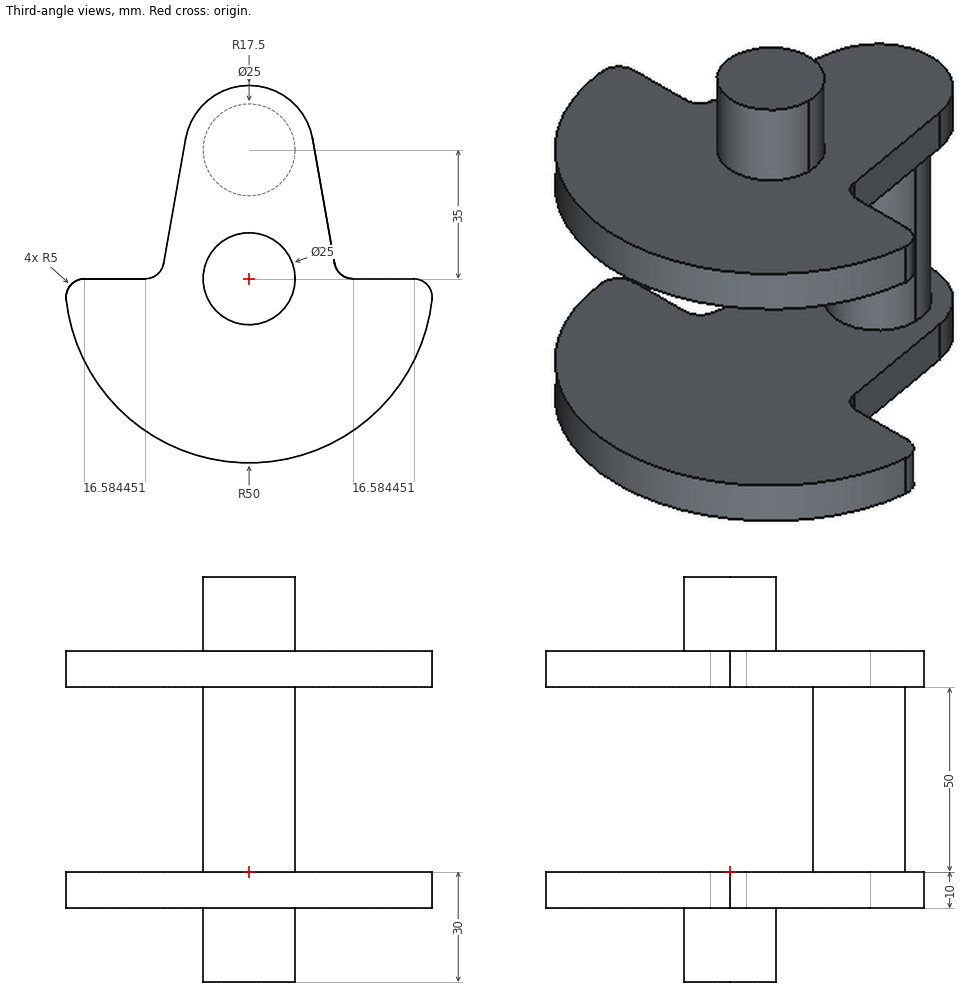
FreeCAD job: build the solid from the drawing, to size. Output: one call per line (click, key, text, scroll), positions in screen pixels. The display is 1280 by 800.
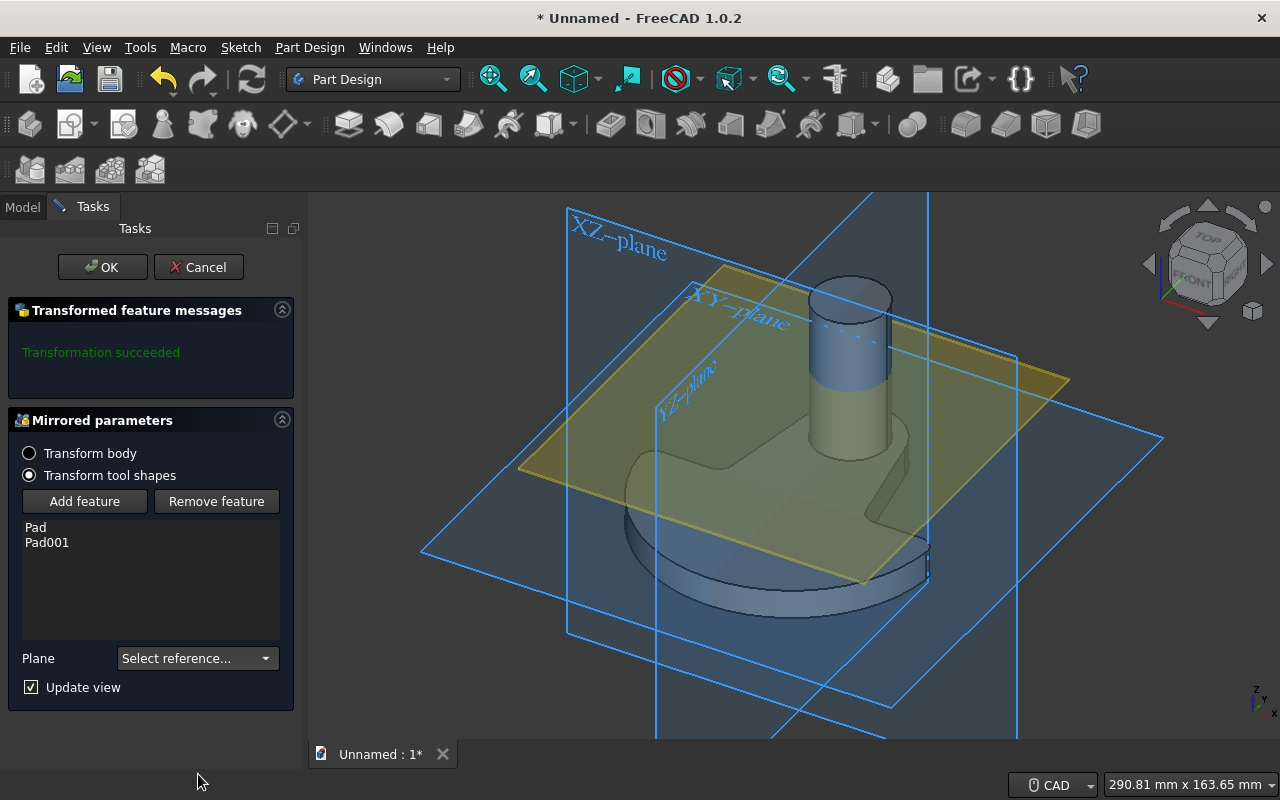
click(23, 206)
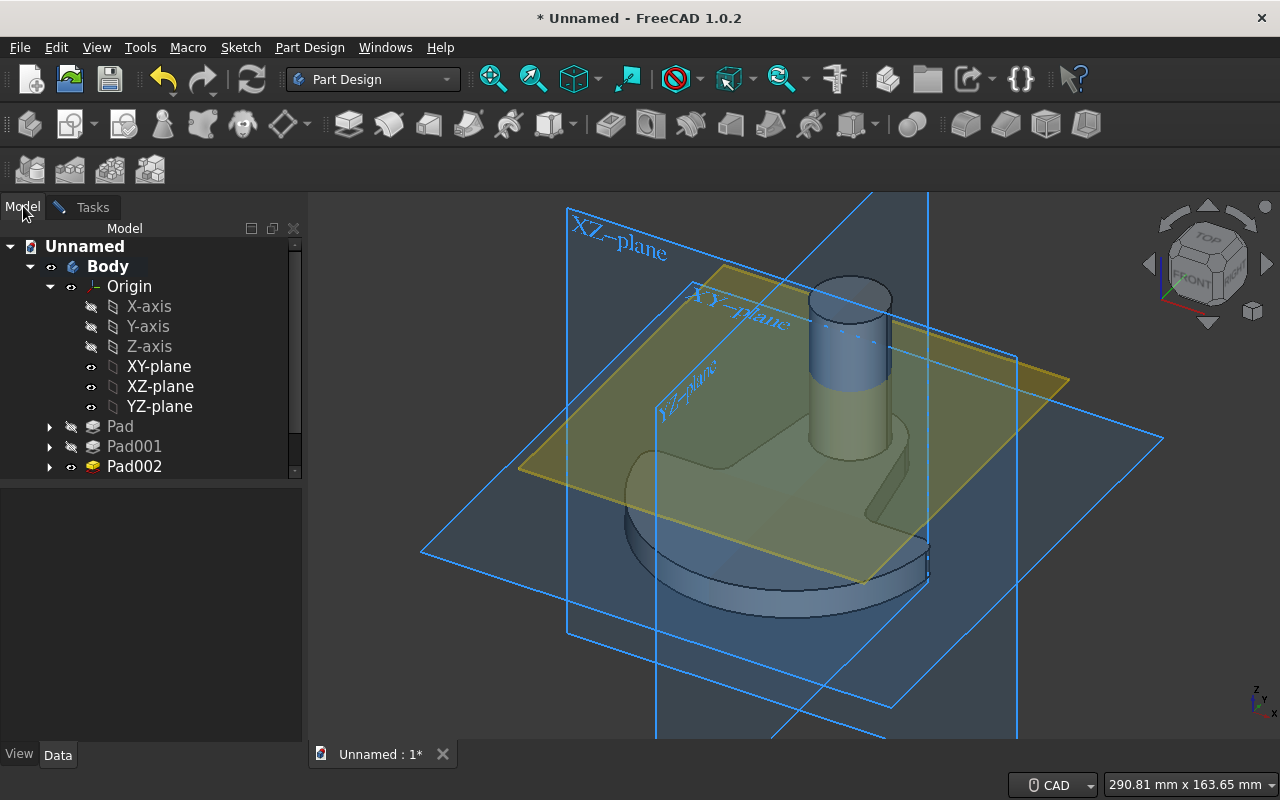
scroll(100, 362, down, 3)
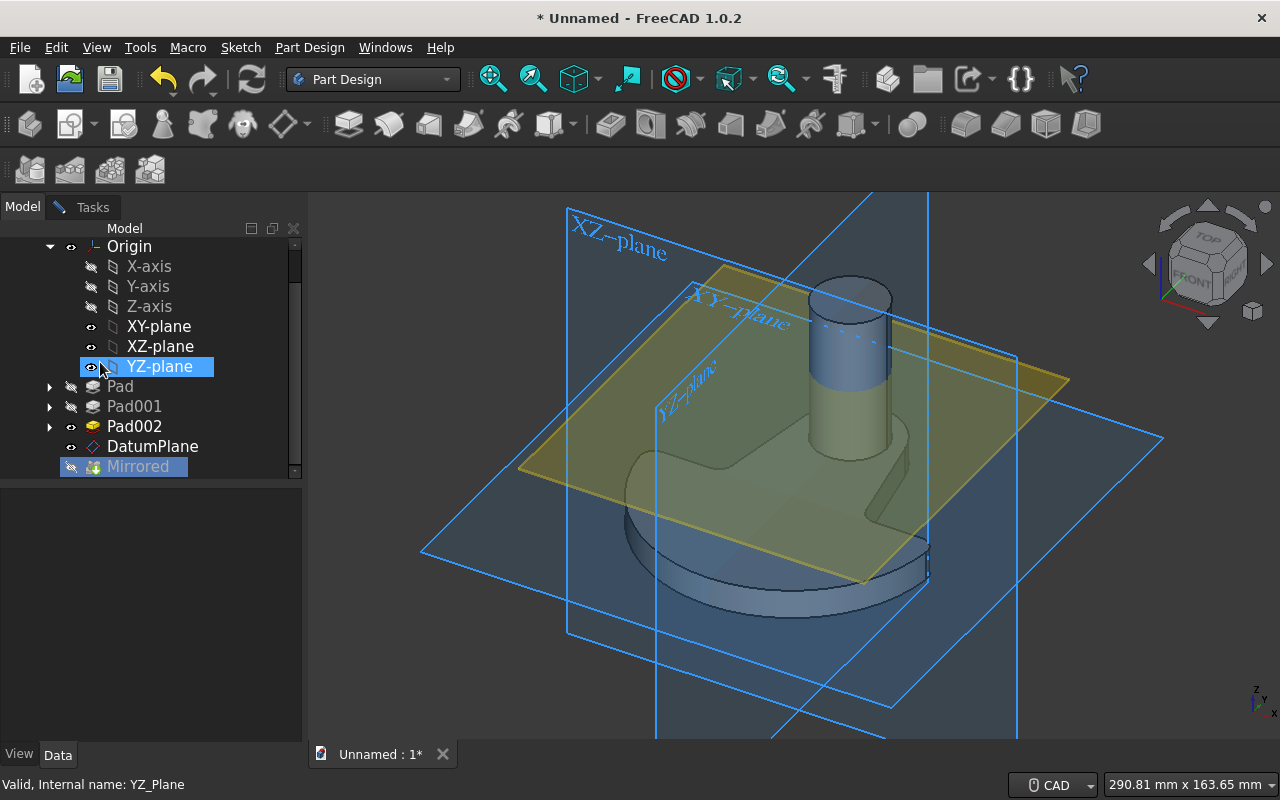
click(116, 447)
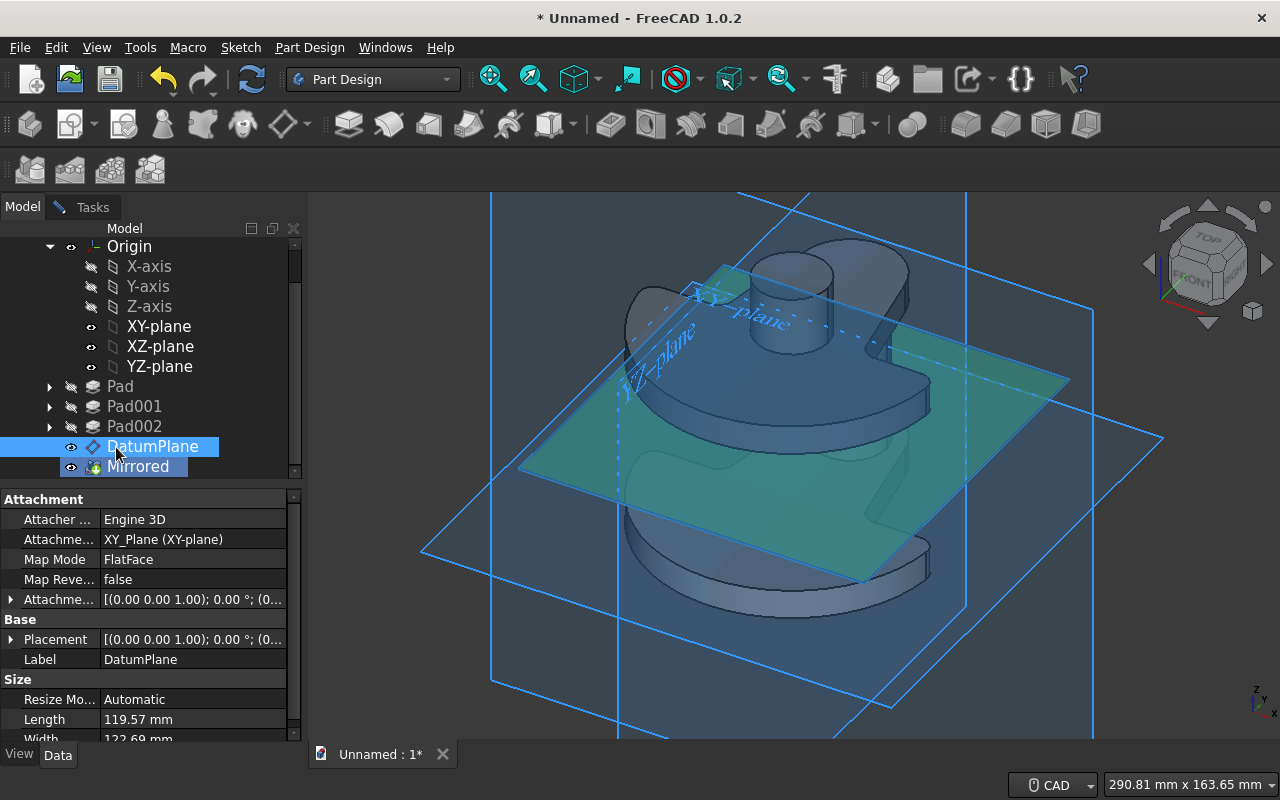
click(84, 206)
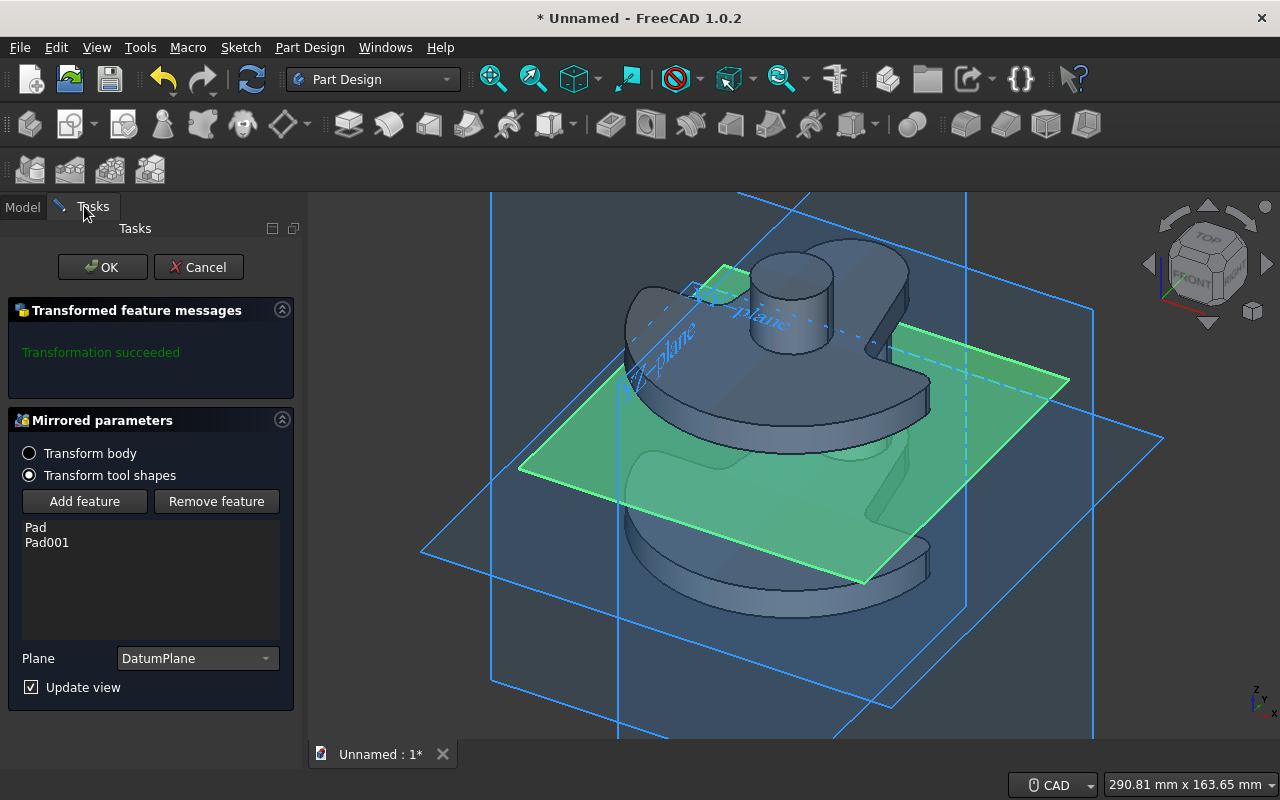
click(103, 267)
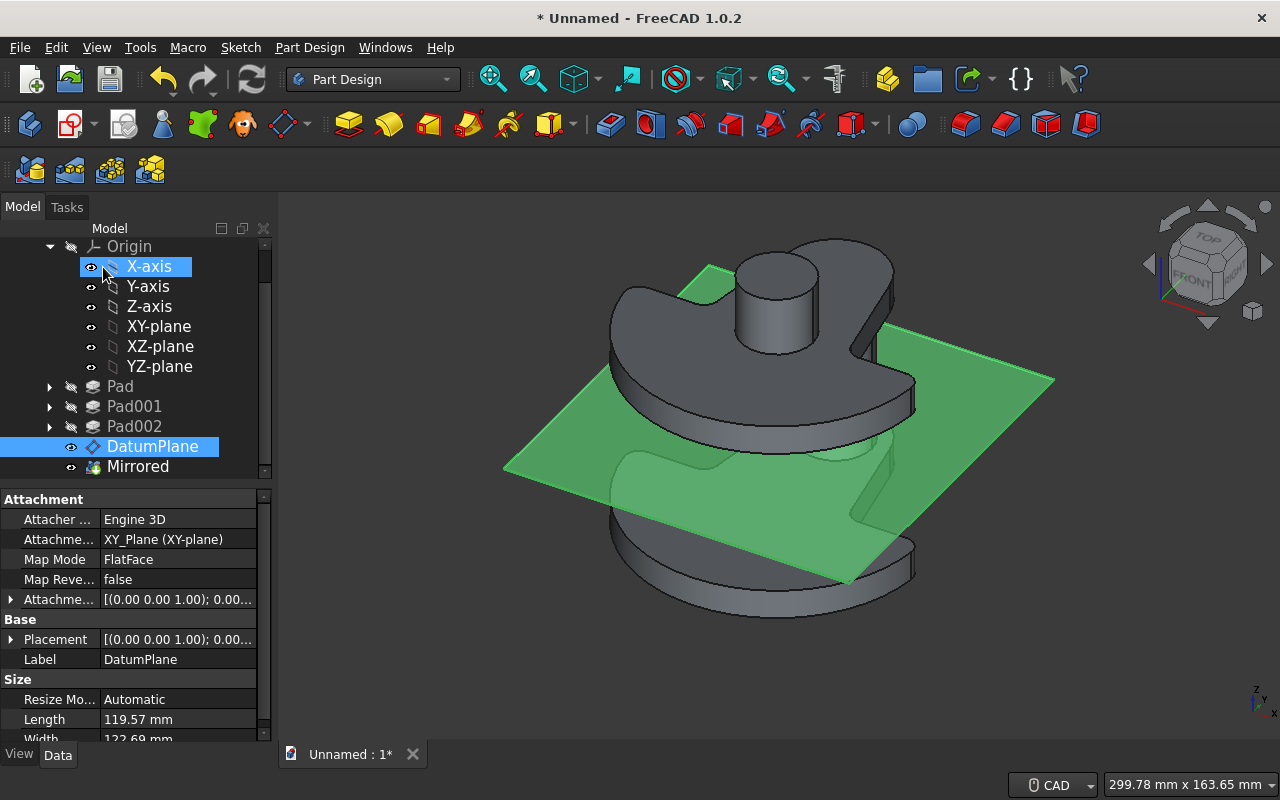
click(116, 447)
key(space)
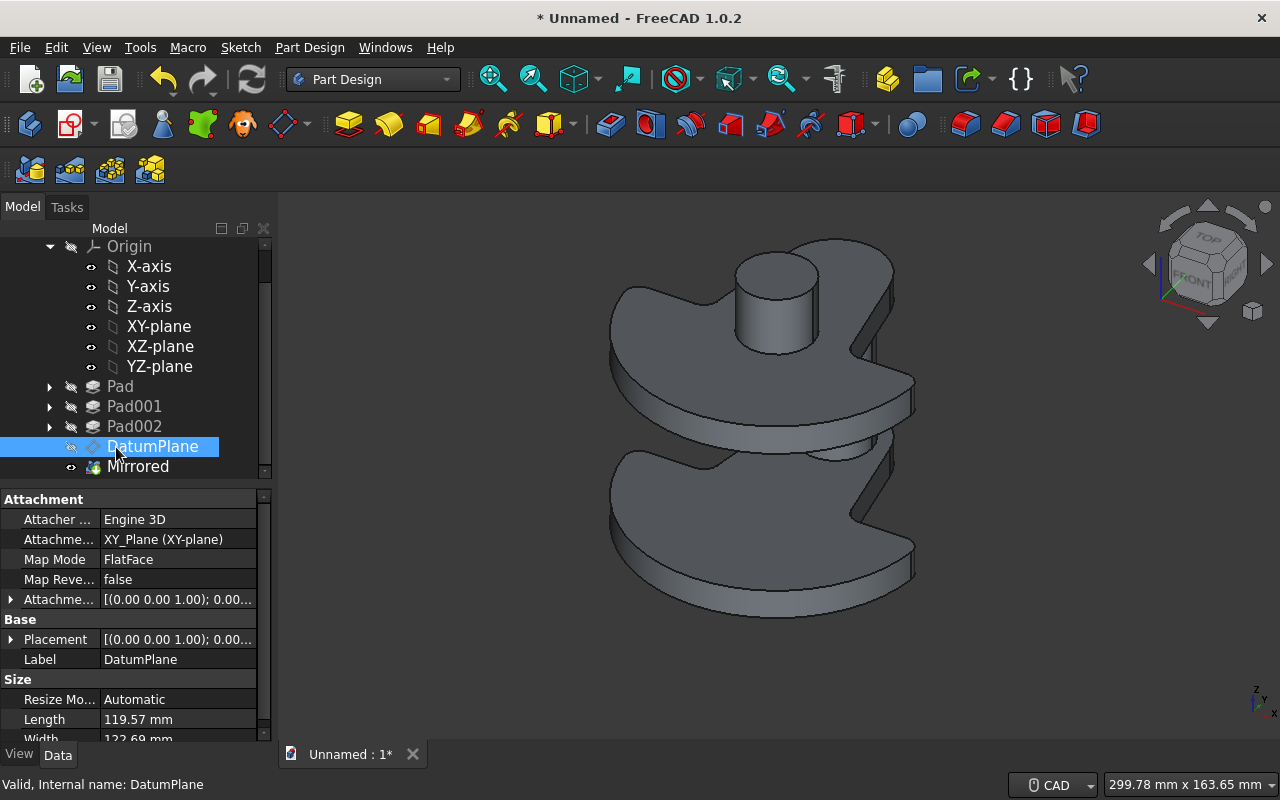
key(0)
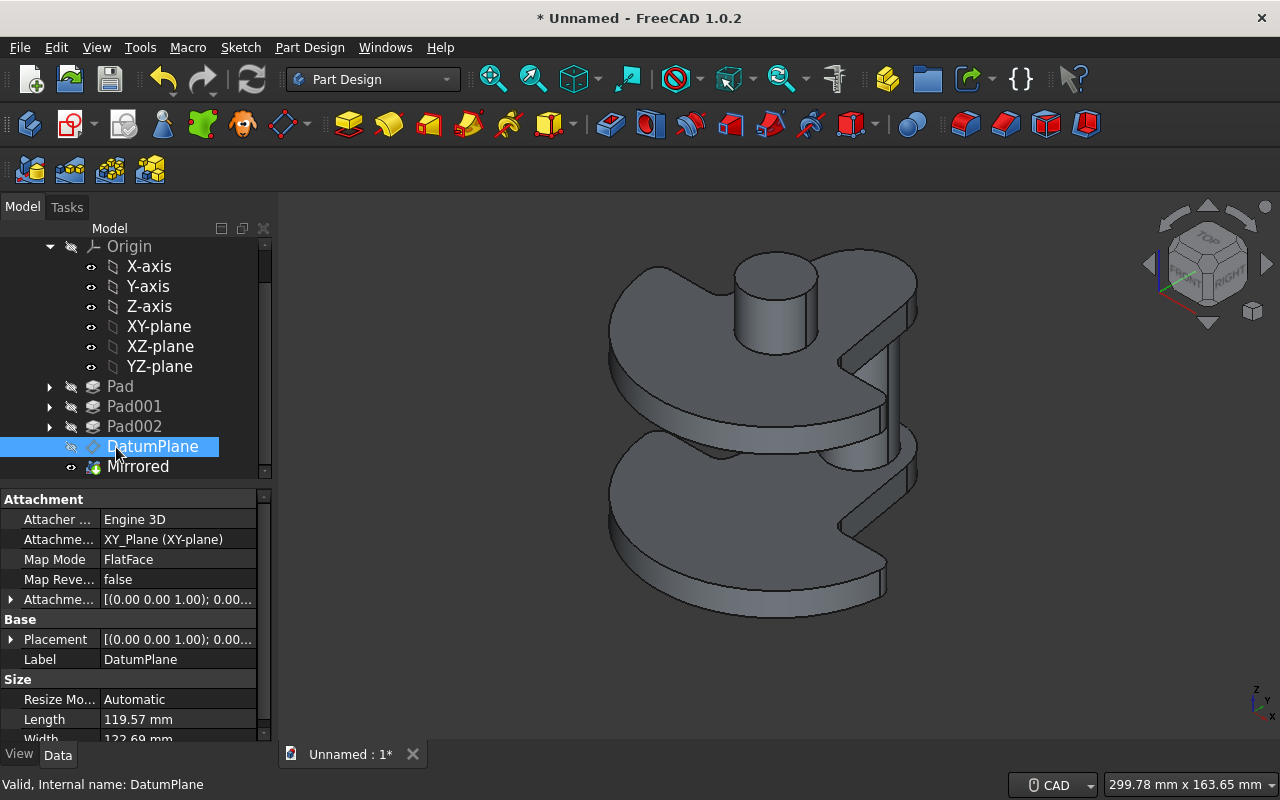
key(v)
key(f)